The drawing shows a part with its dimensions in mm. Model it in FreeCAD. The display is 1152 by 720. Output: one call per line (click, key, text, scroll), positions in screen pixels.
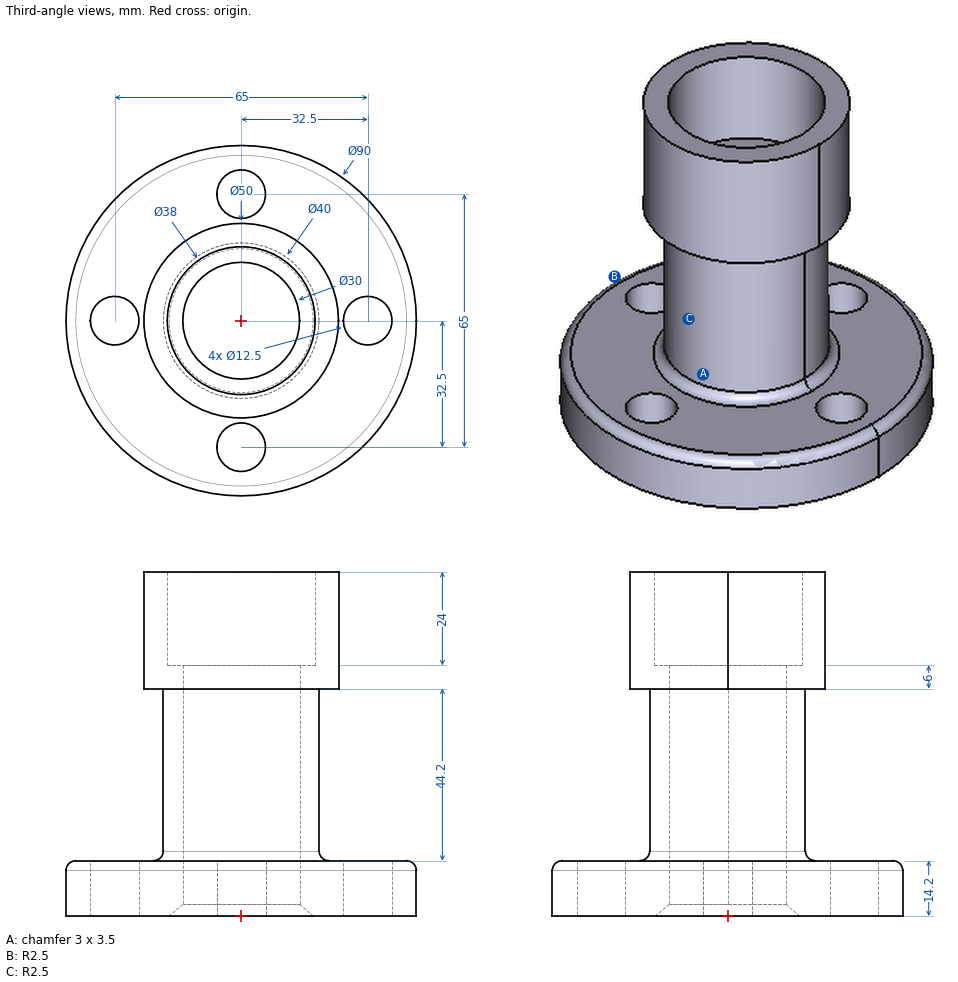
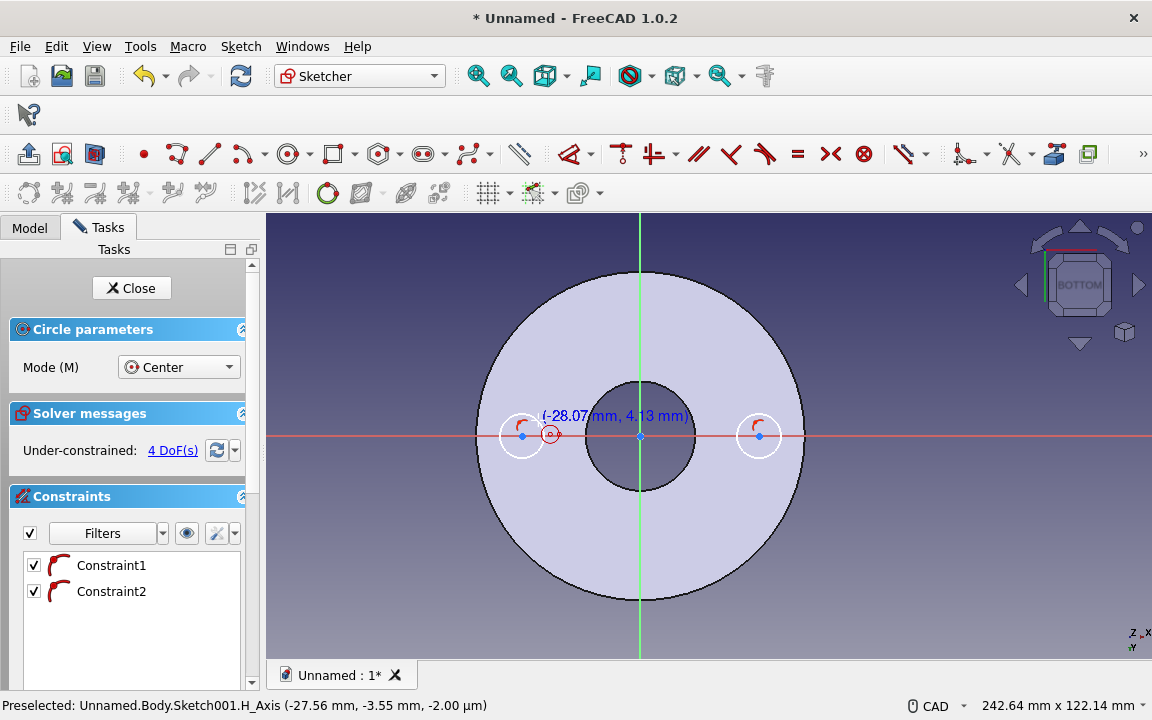
click(640, 317)
click(657, 301)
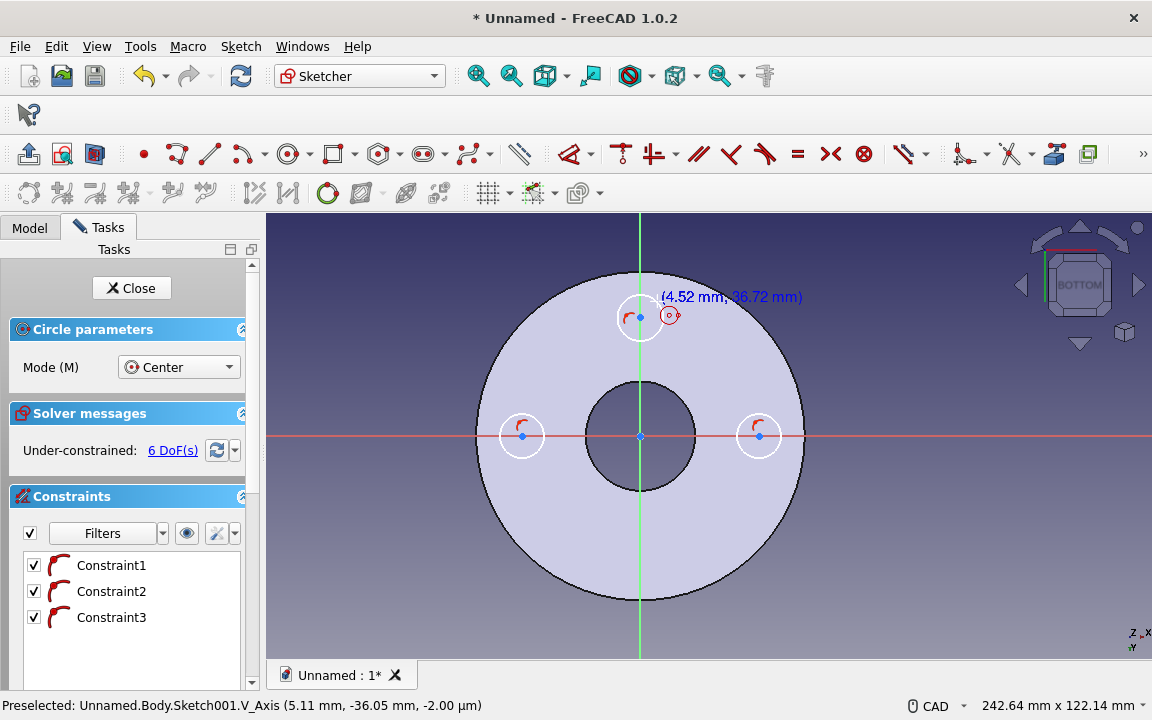
click(640, 555)
click(657, 539)
key(Escape)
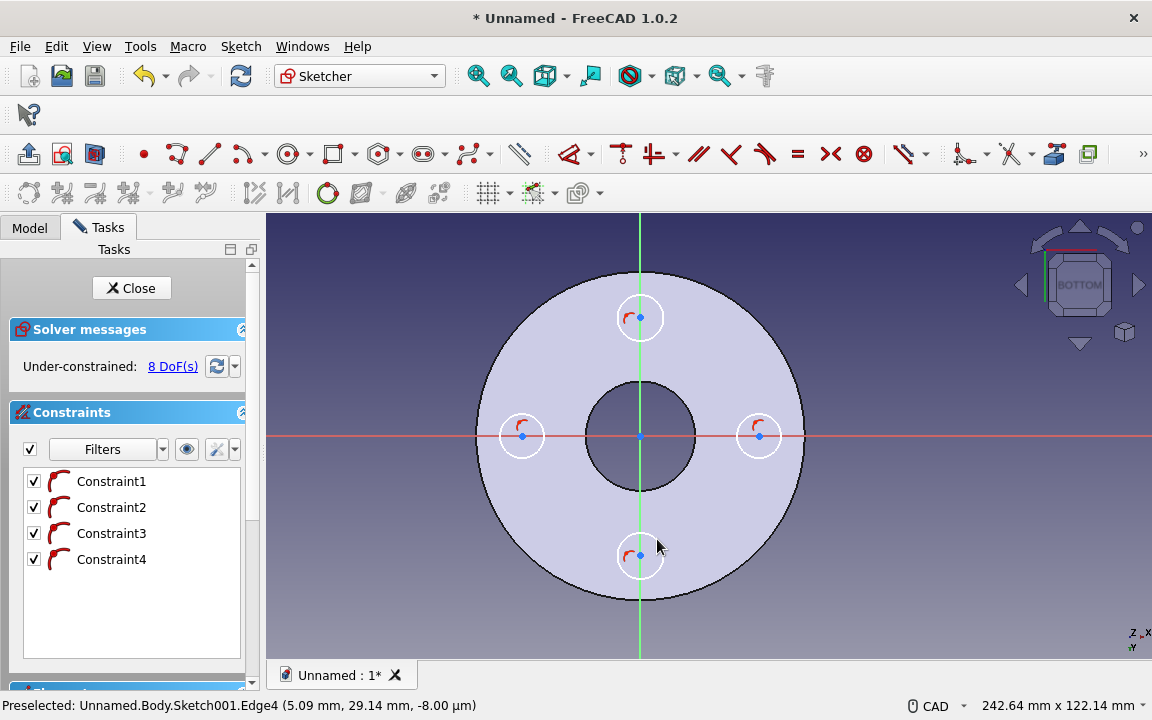
click(775, 420)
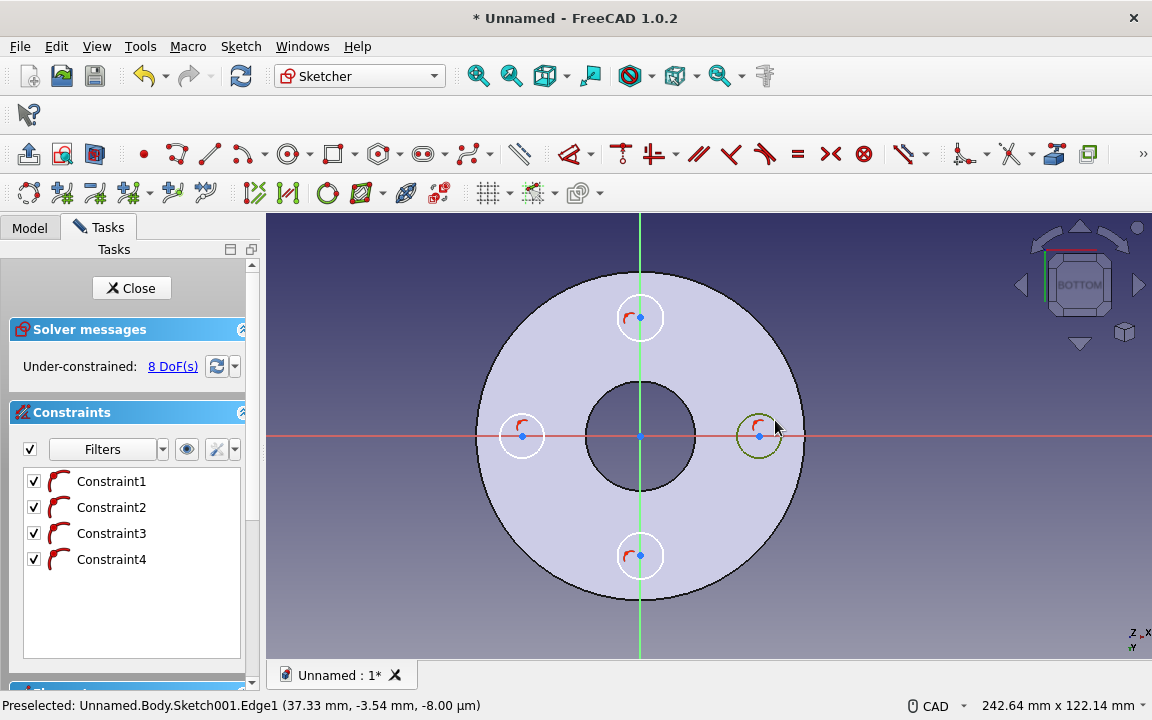
click(538, 420)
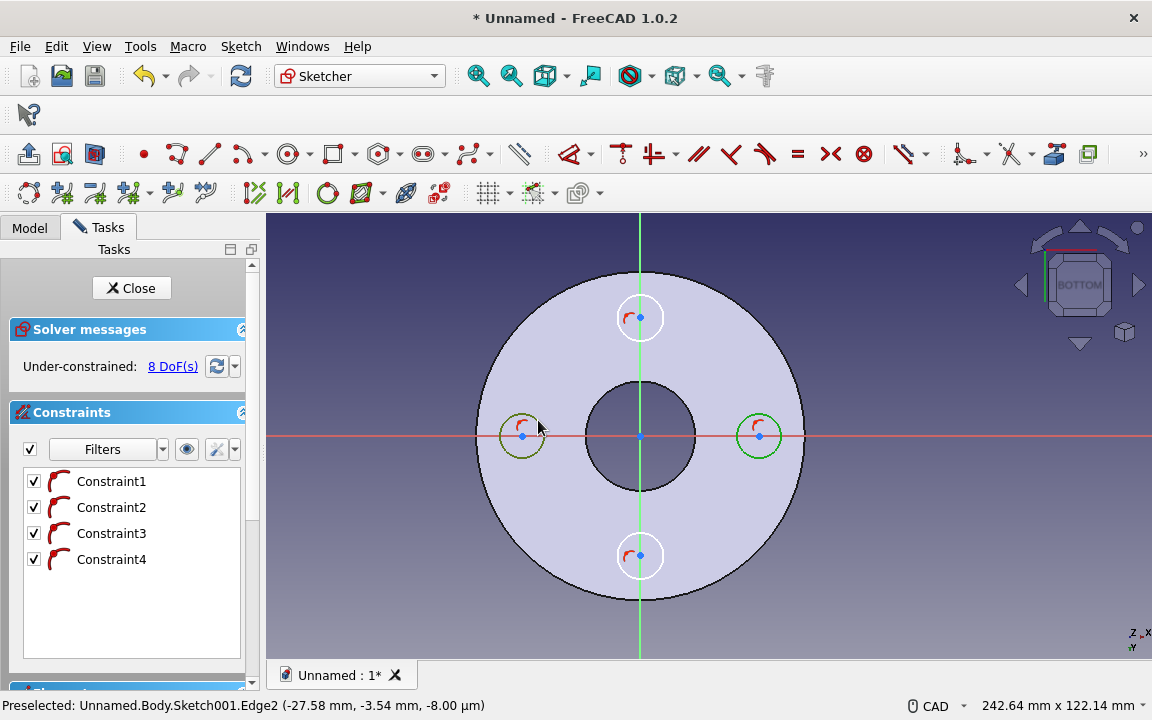
click(657, 302)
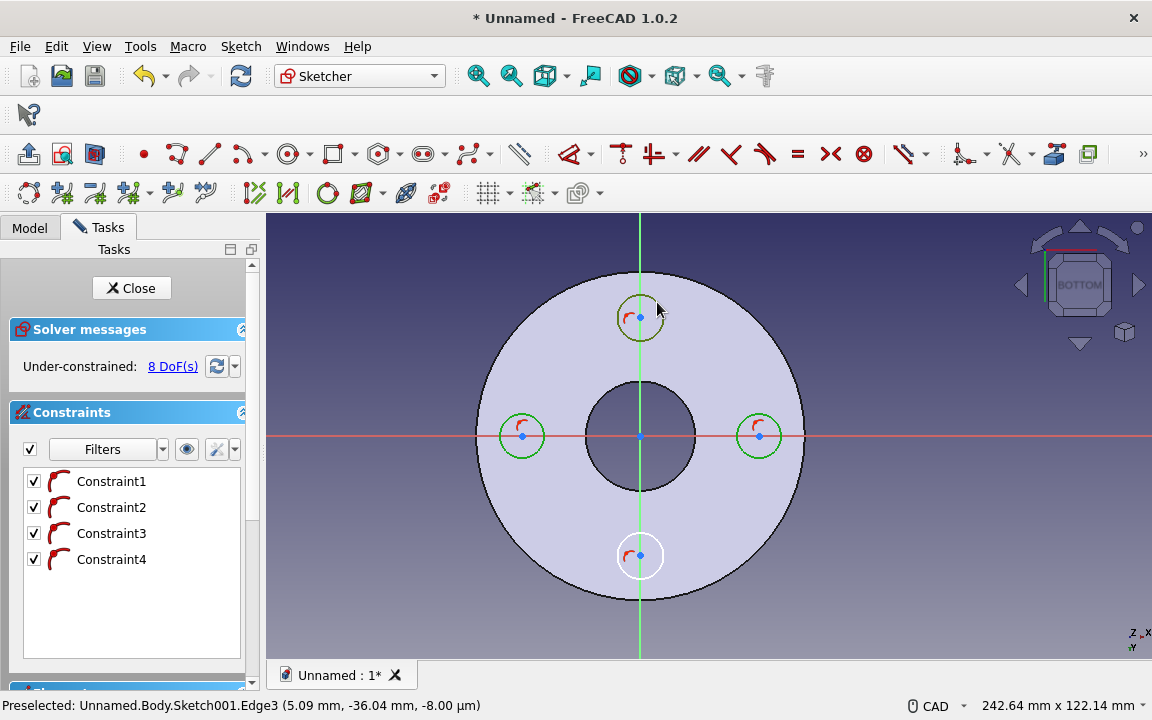
click(657, 540)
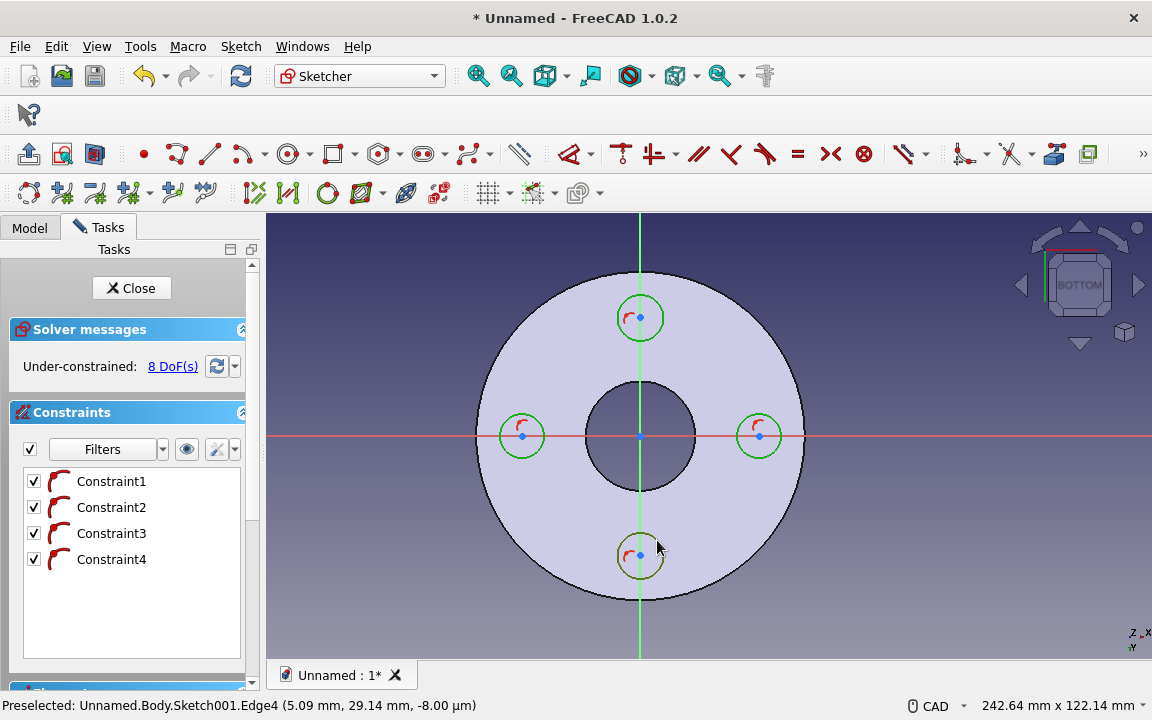
click(798, 154)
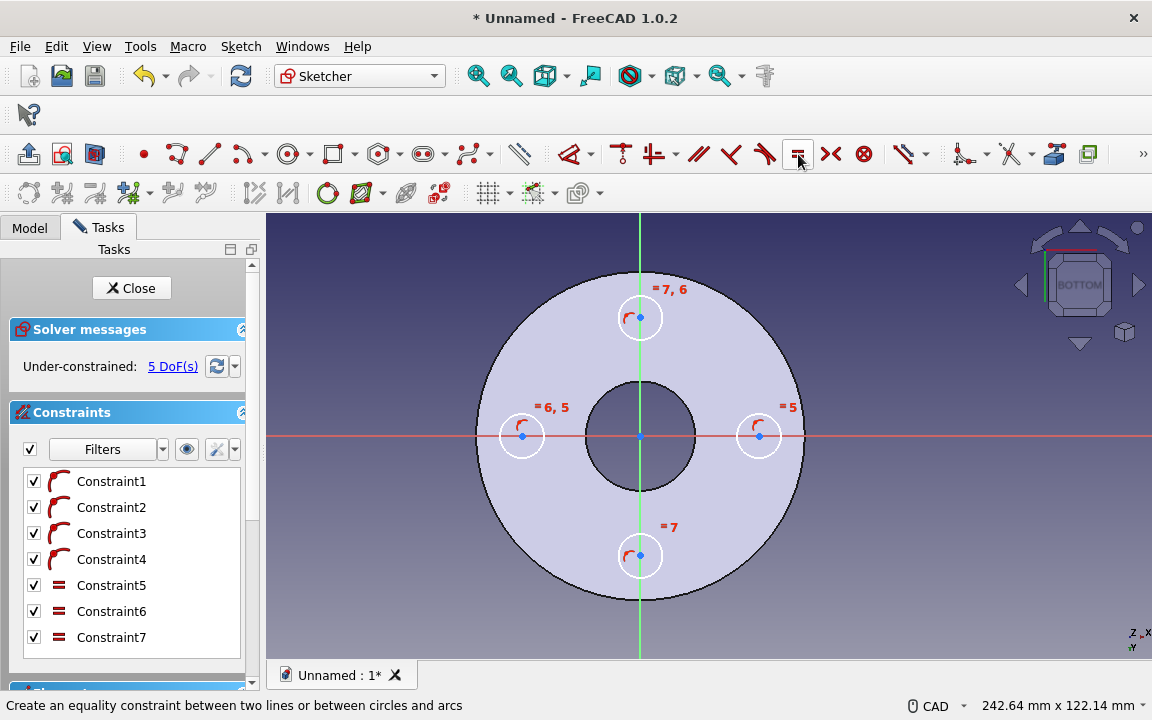
click(568, 154)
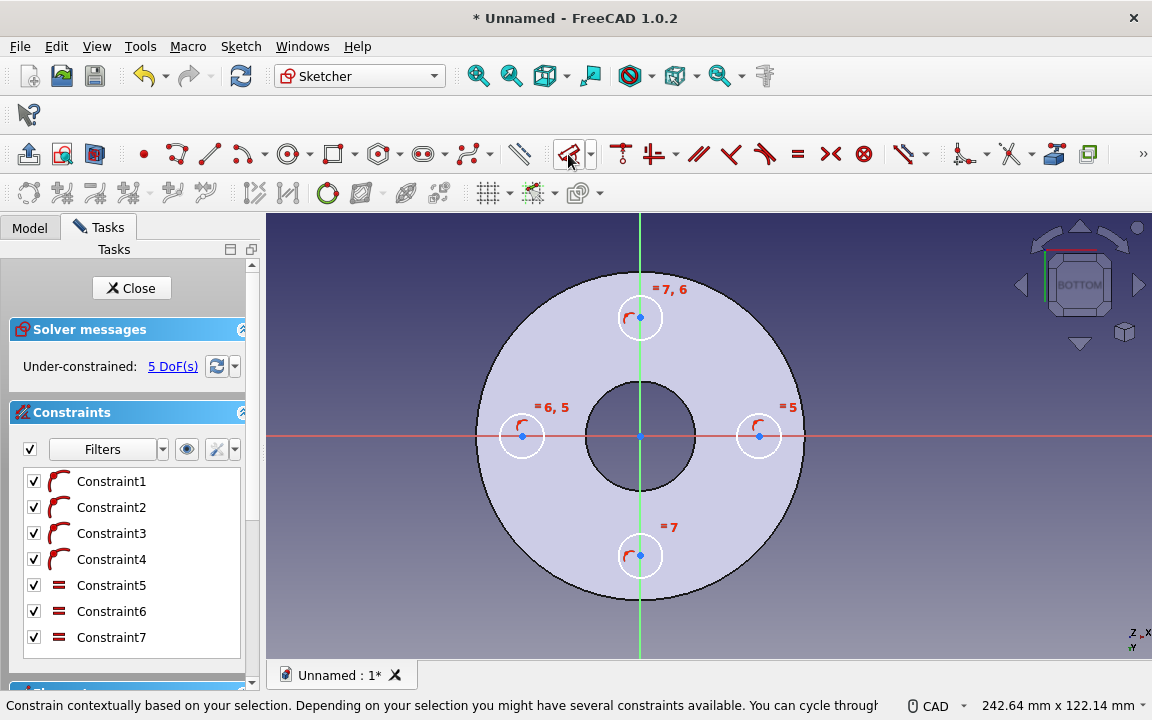
click(775, 420)
click(798, 397)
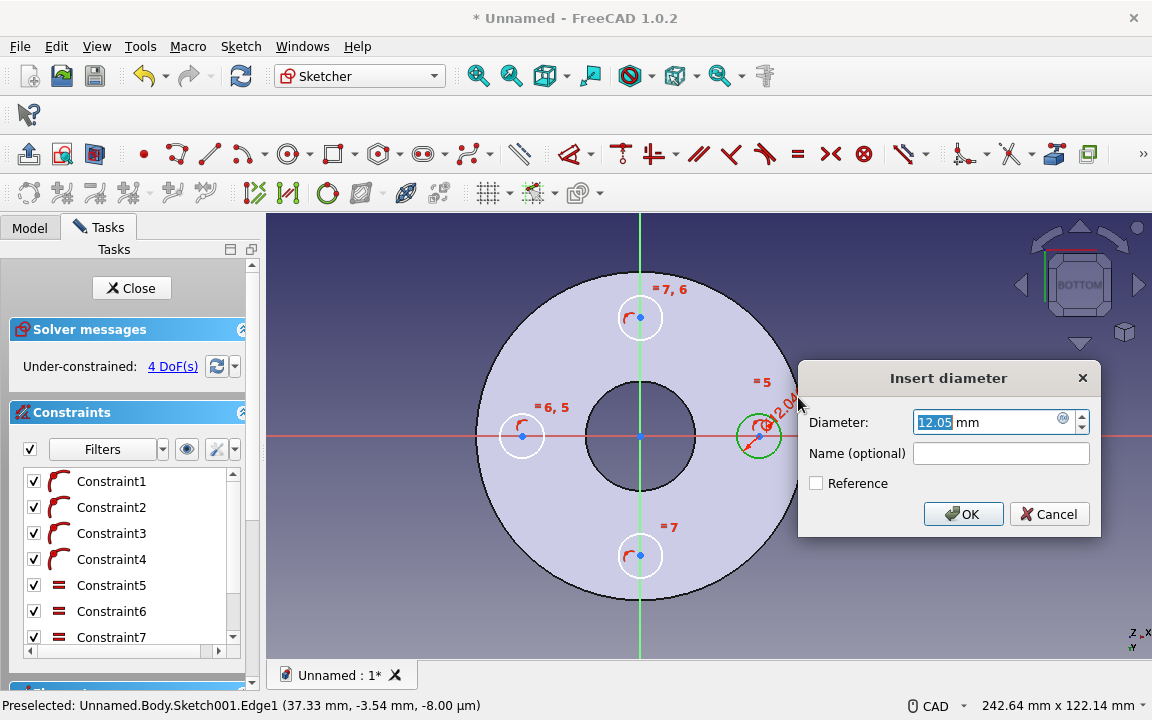
text(12.5)
key(Return)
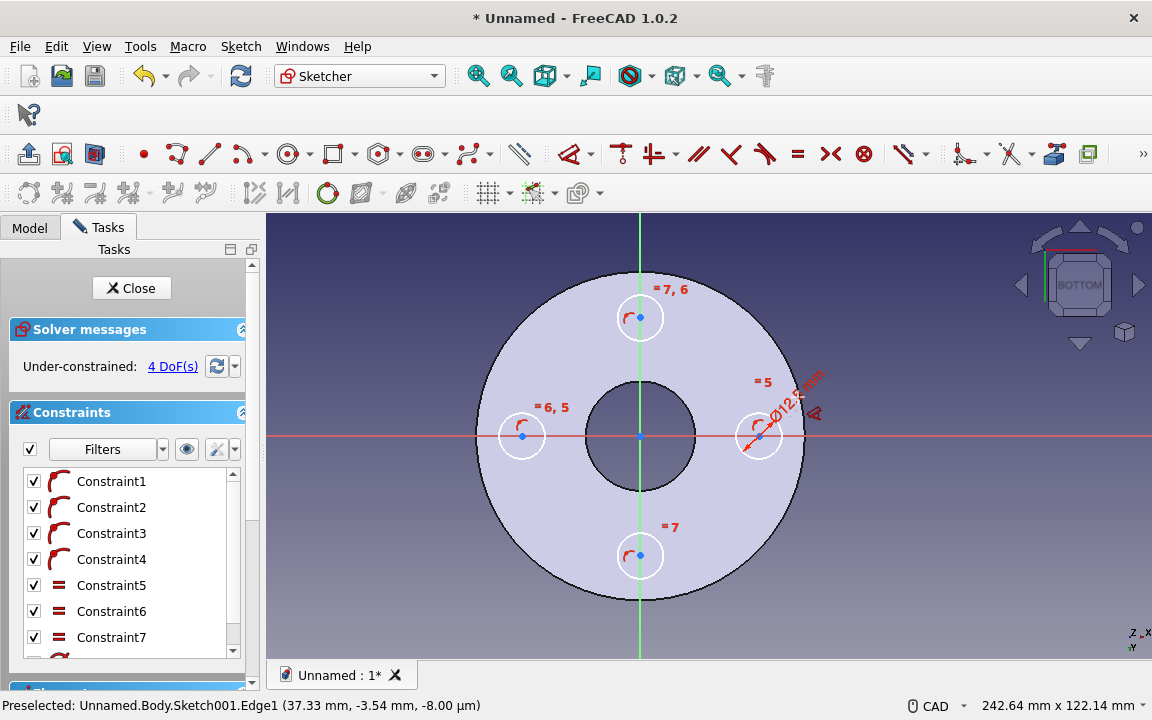
click(759, 436)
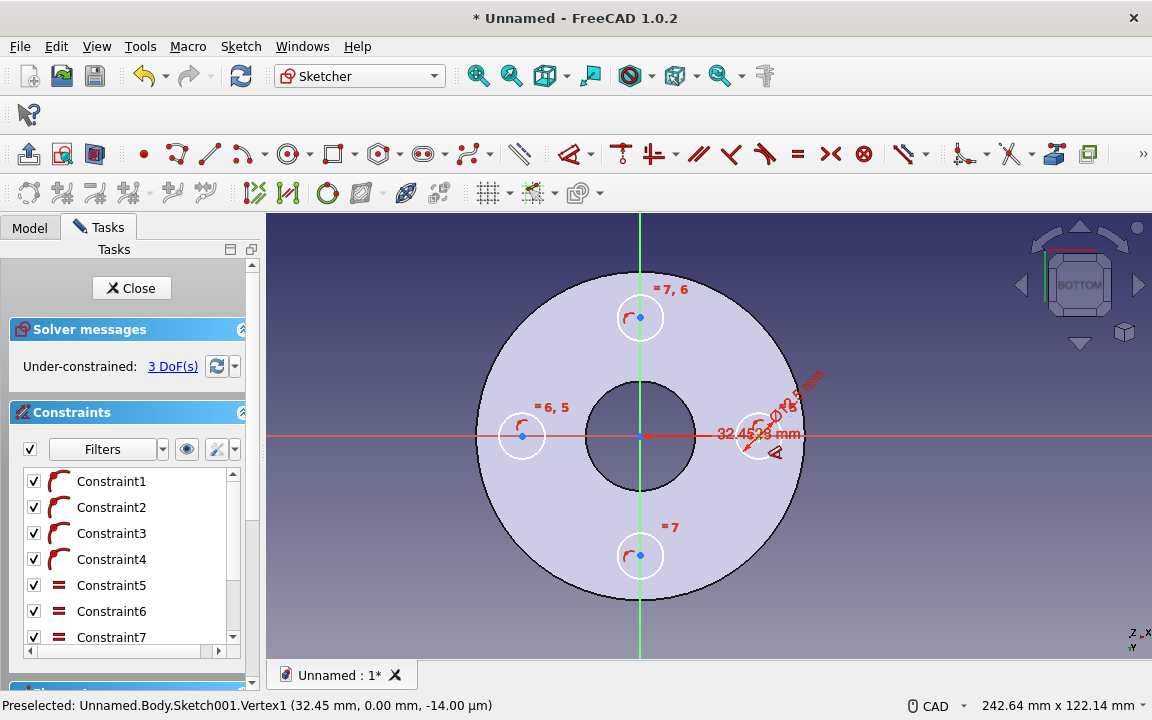
click(522, 436)
click(586, 470)